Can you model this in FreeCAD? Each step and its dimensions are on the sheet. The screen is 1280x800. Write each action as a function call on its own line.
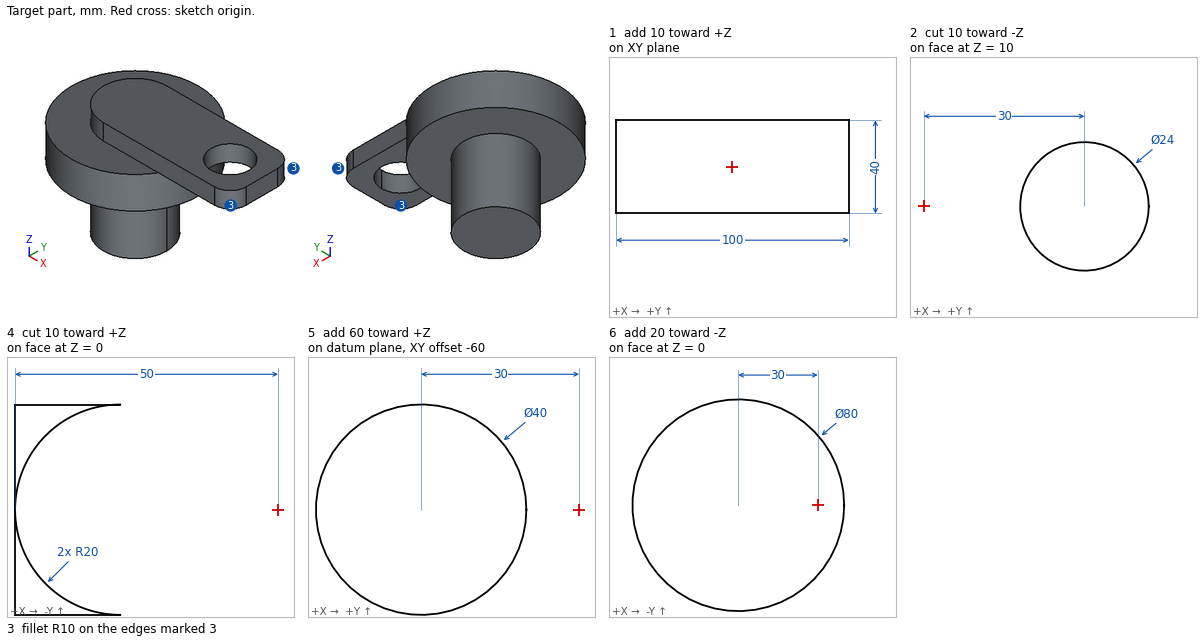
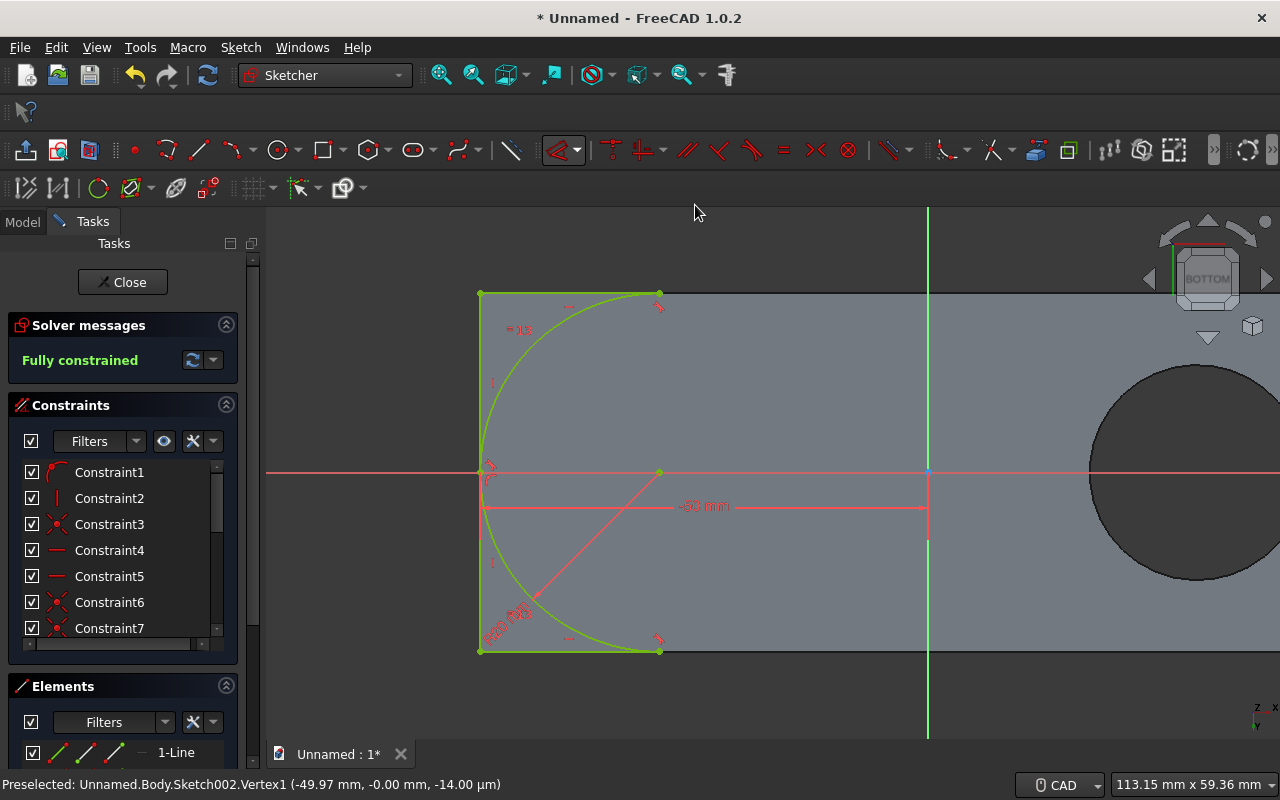
click(123, 282)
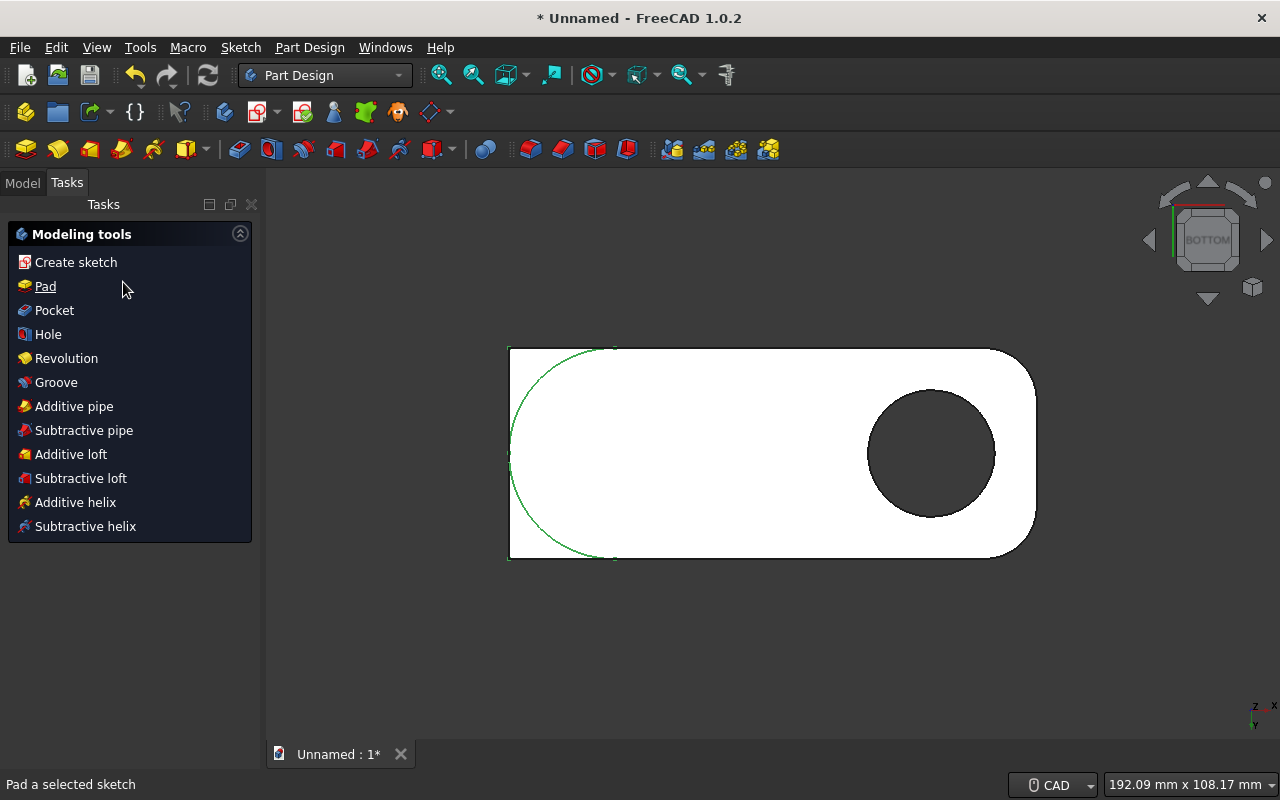
click(240, 150)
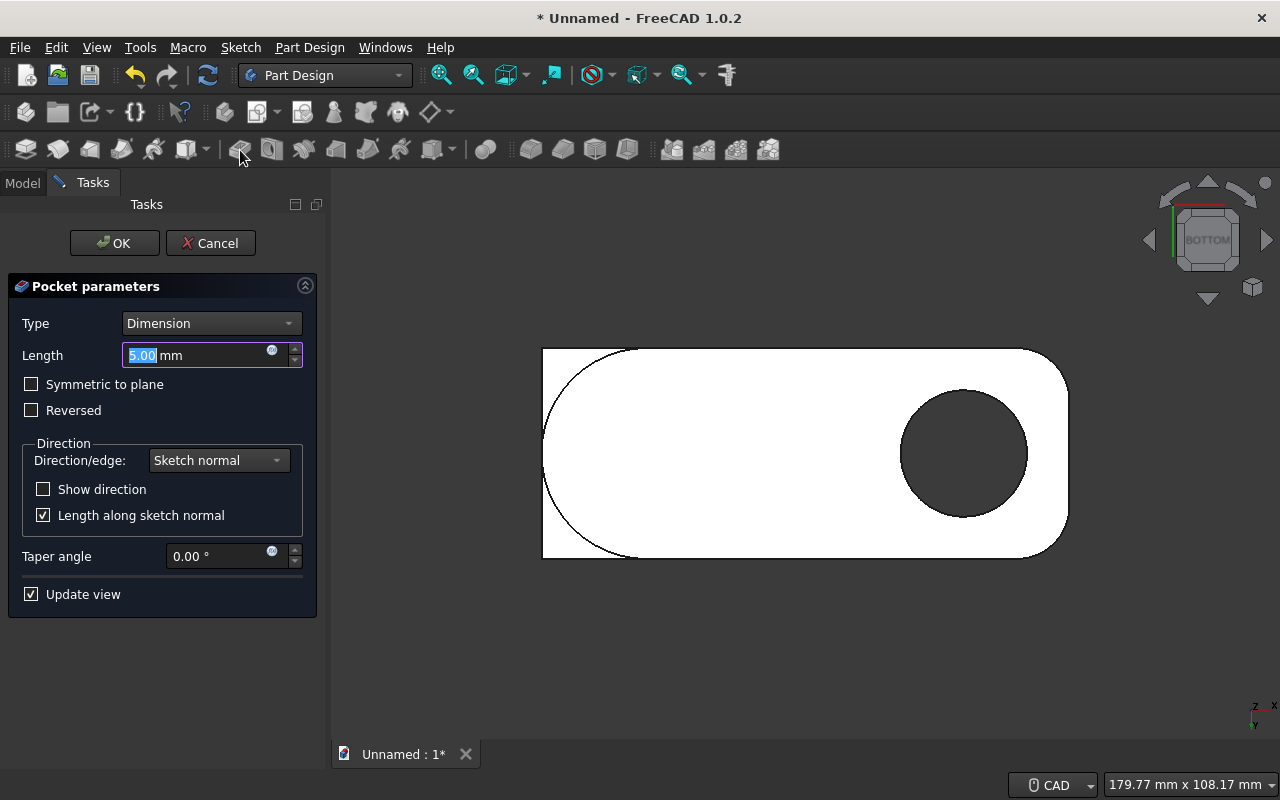
text(10)
key(Tab)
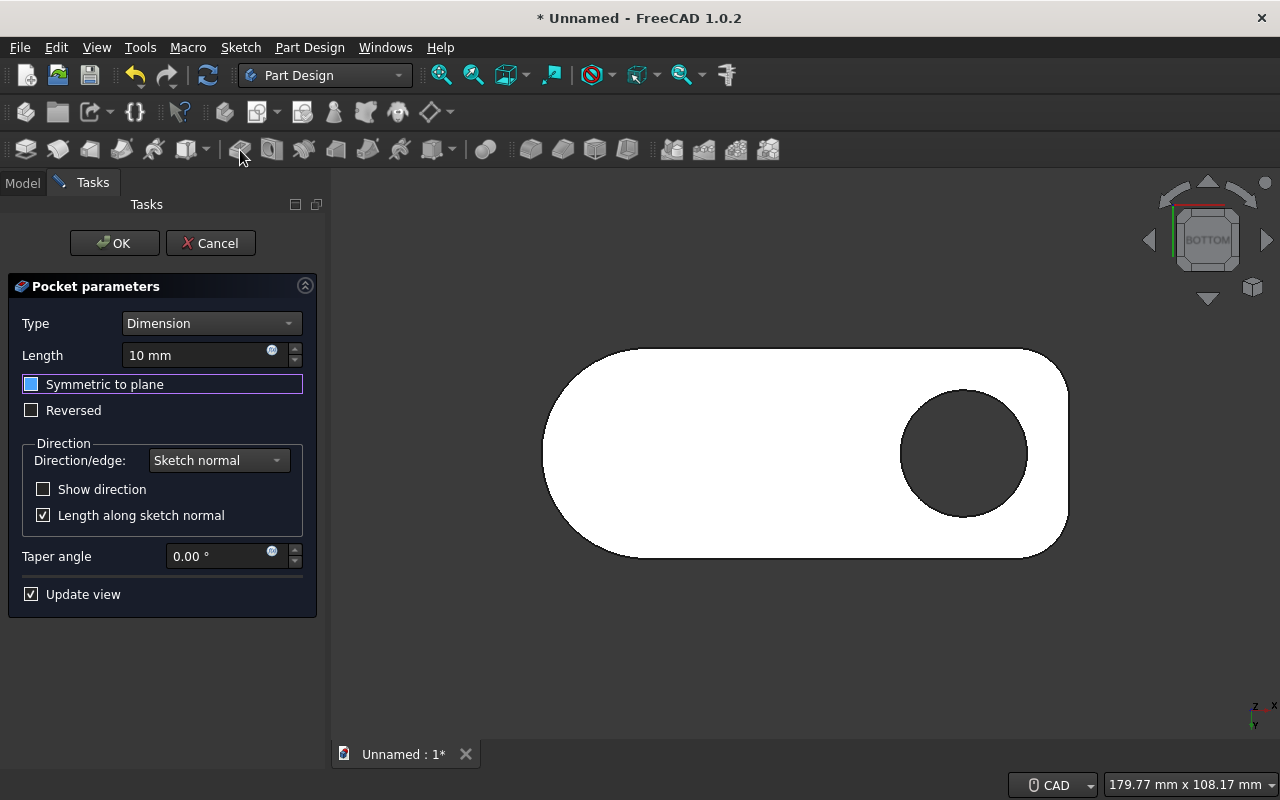
click(115, 243)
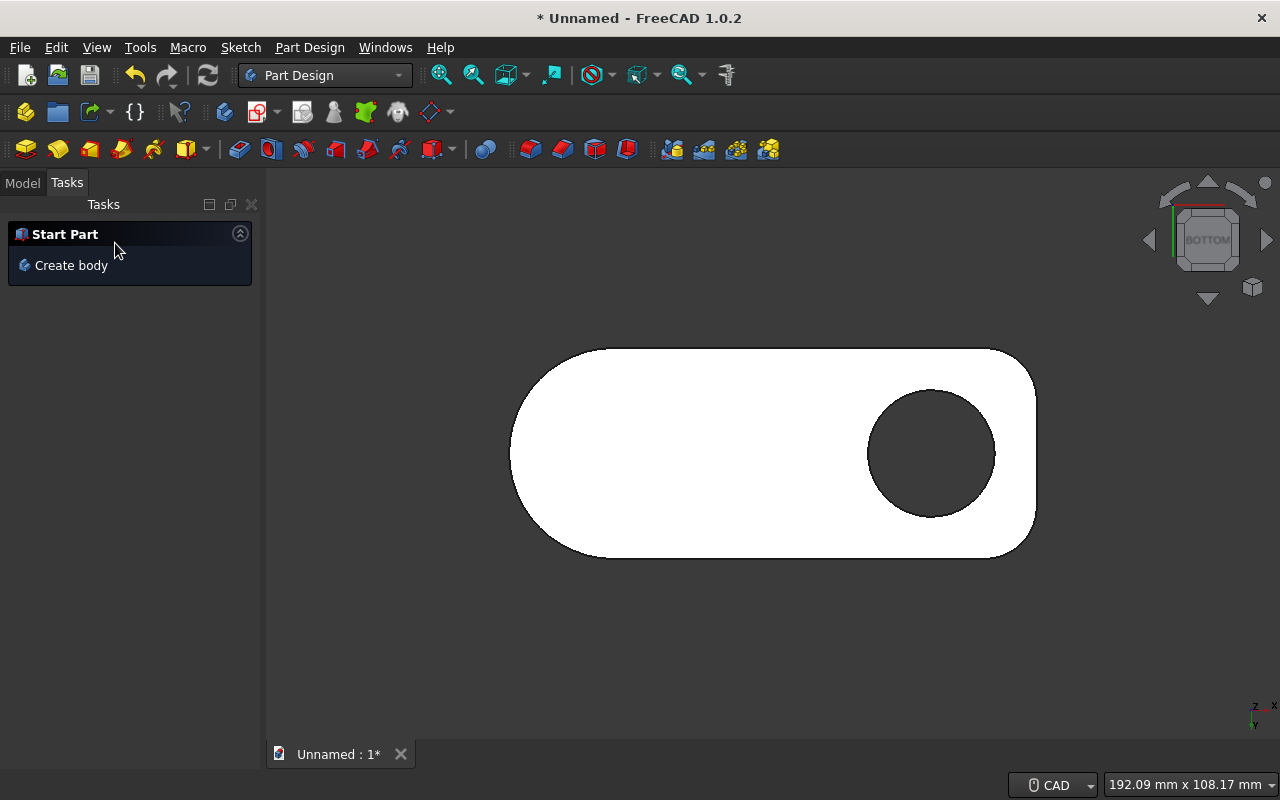
click(23, 182)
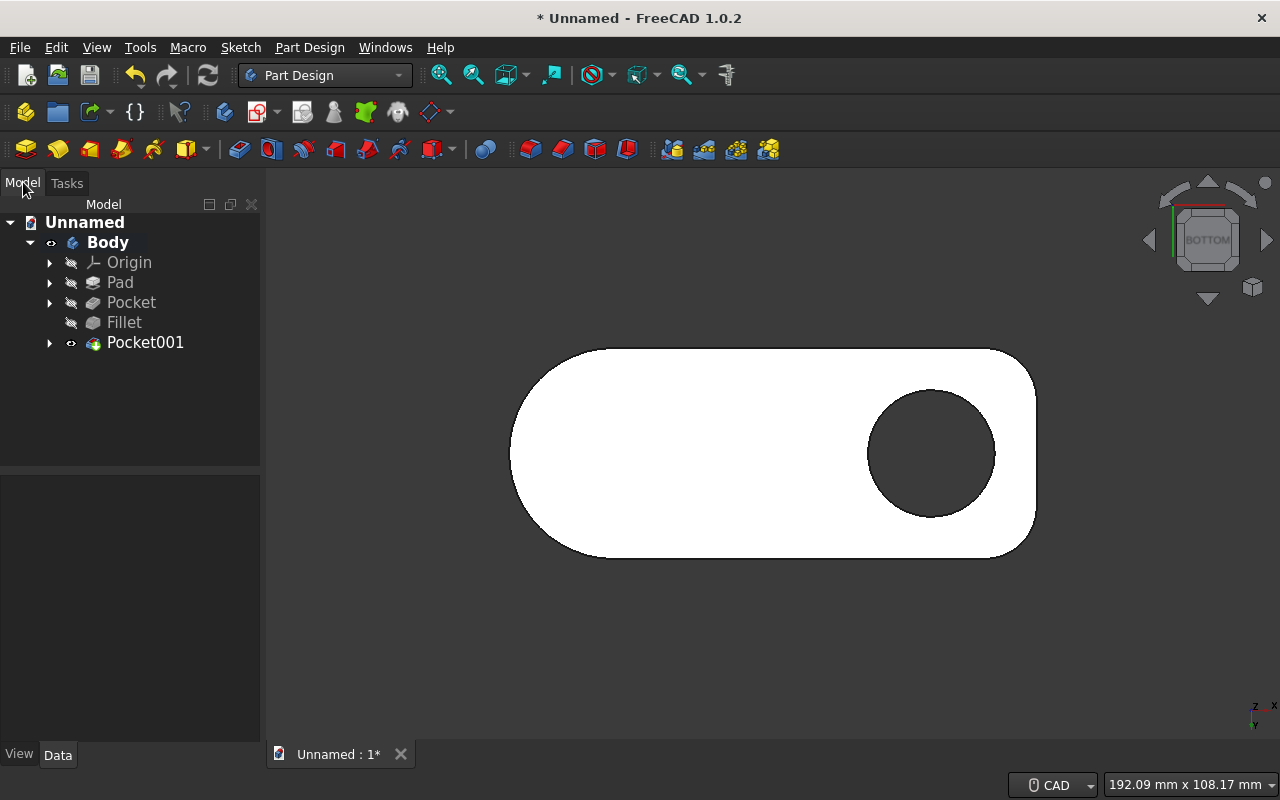
click(50, 263)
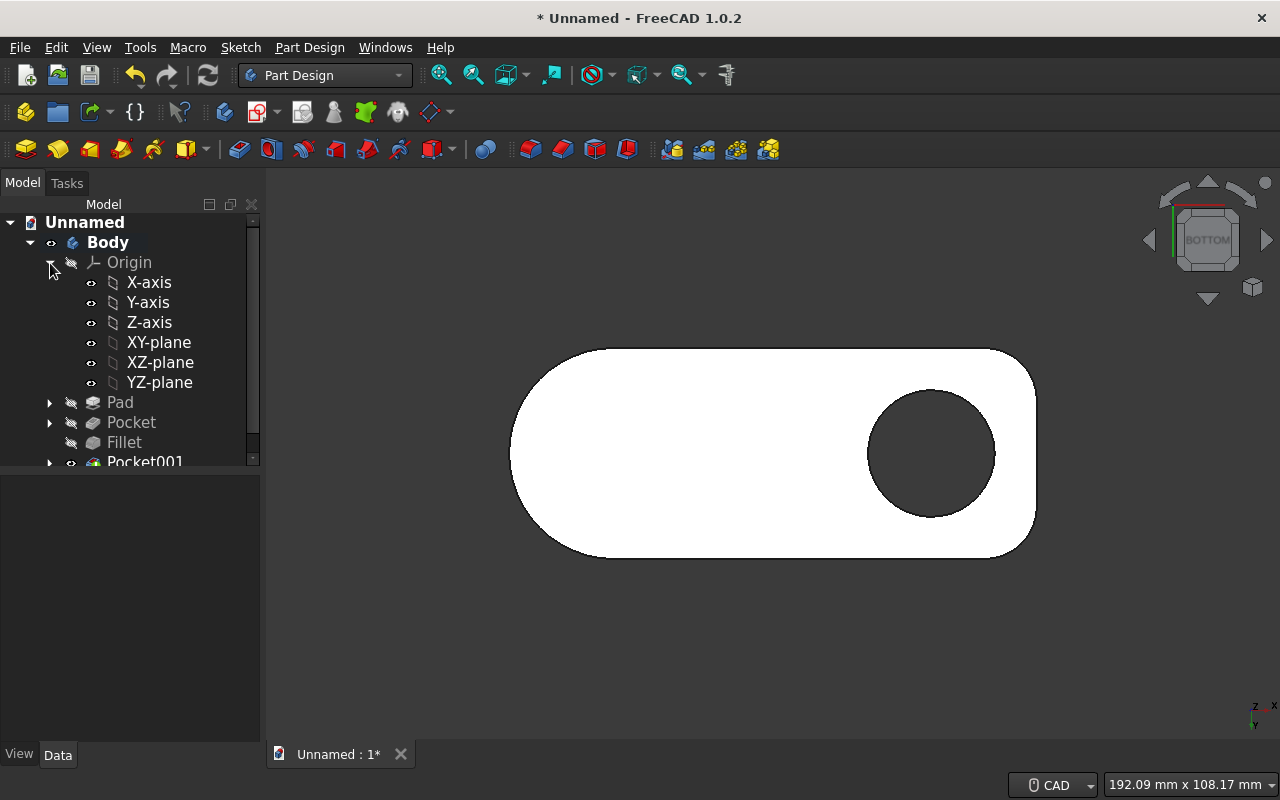
click(136, 343)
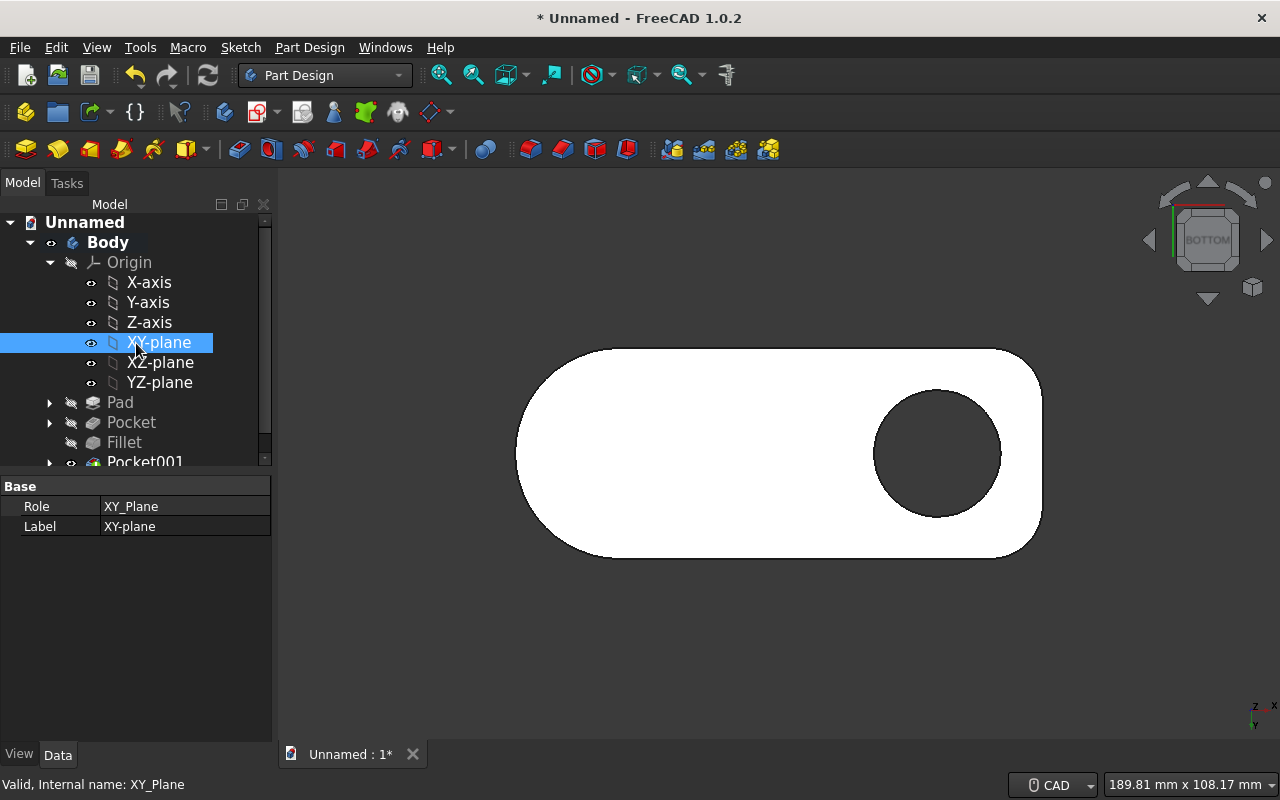
click(430, 112)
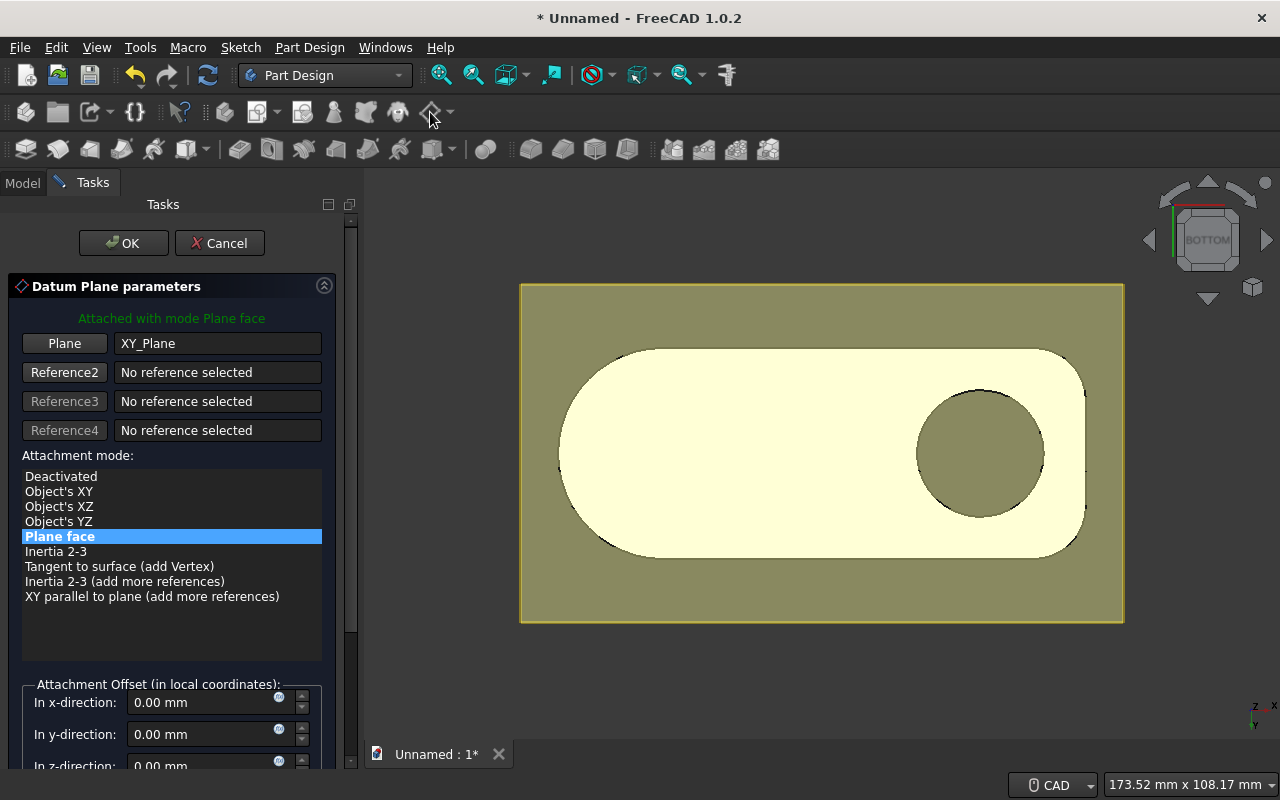
scroll(351, 491, down, 2)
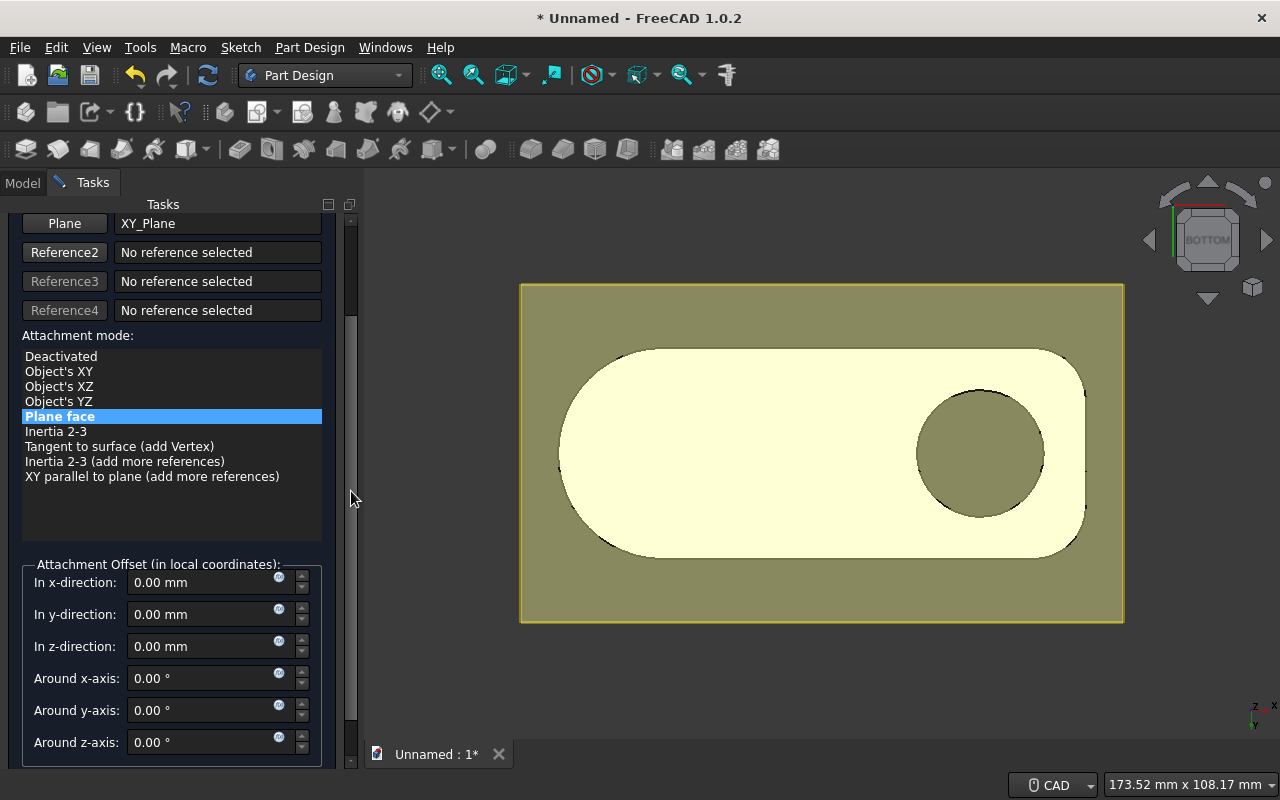
triple_click(210, 646)